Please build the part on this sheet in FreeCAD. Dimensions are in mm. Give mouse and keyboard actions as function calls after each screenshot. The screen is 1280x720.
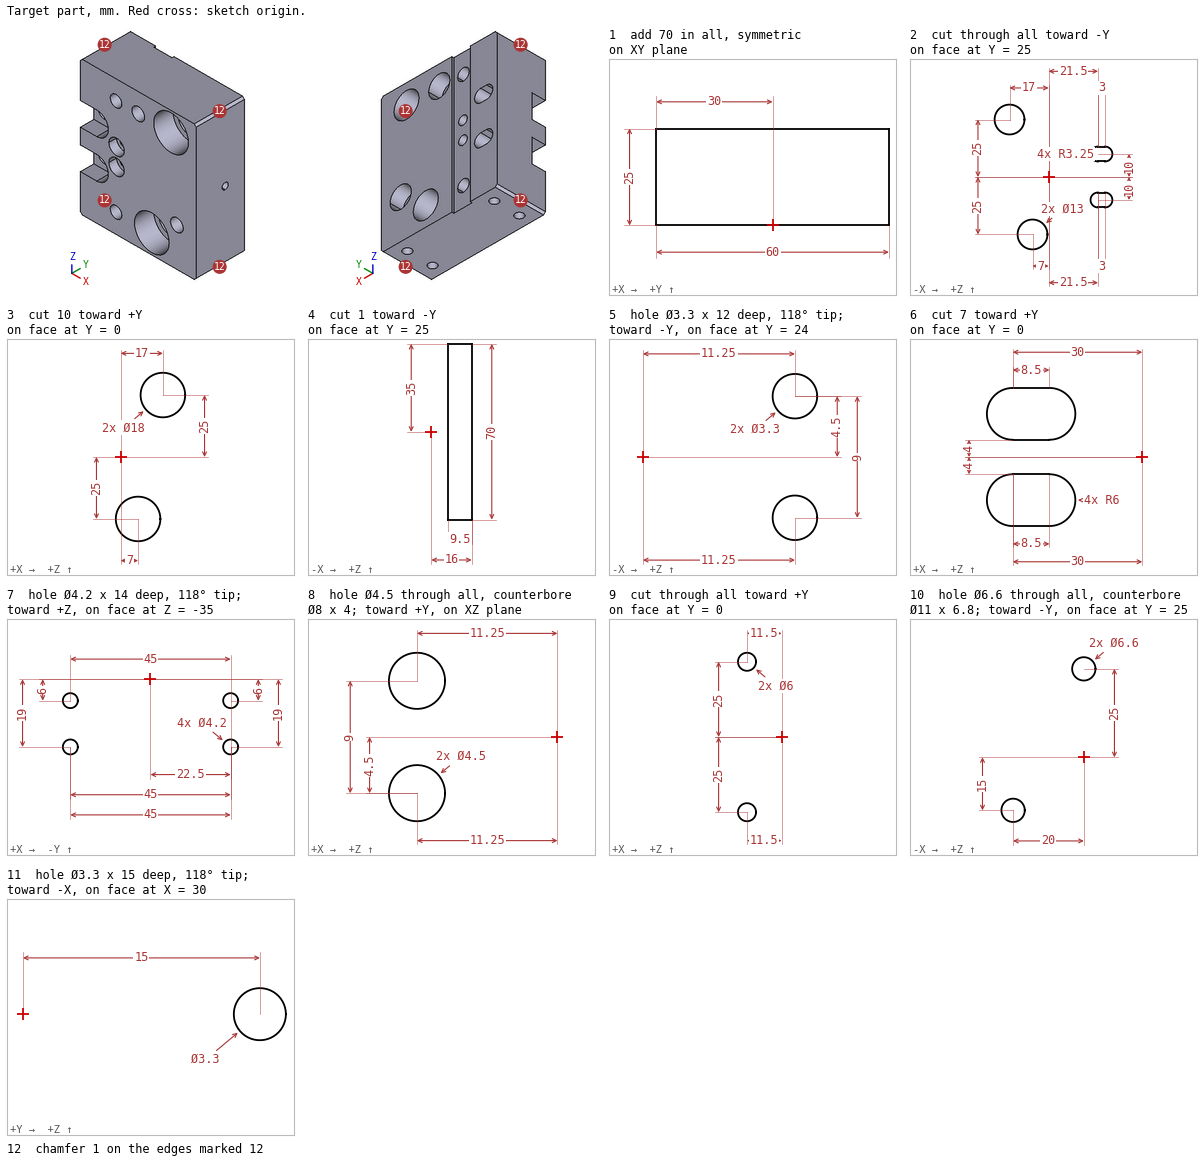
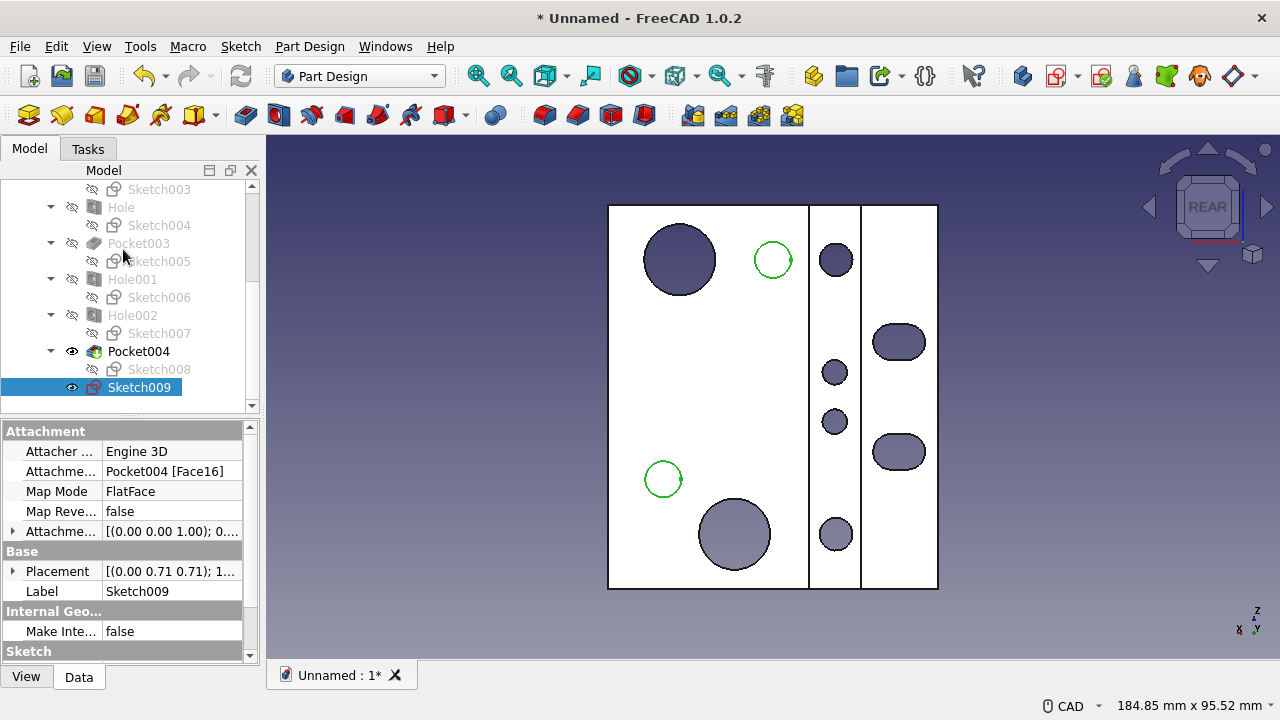
click(279, 116)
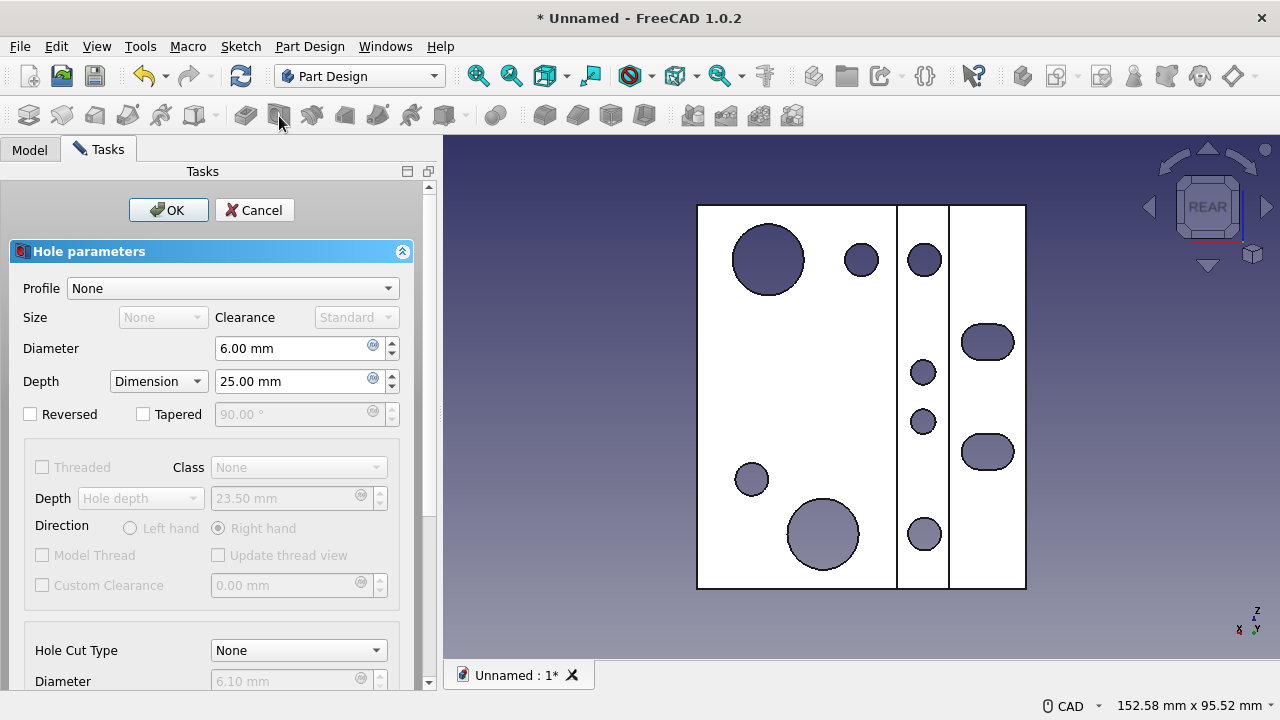
triple_click(300, 348)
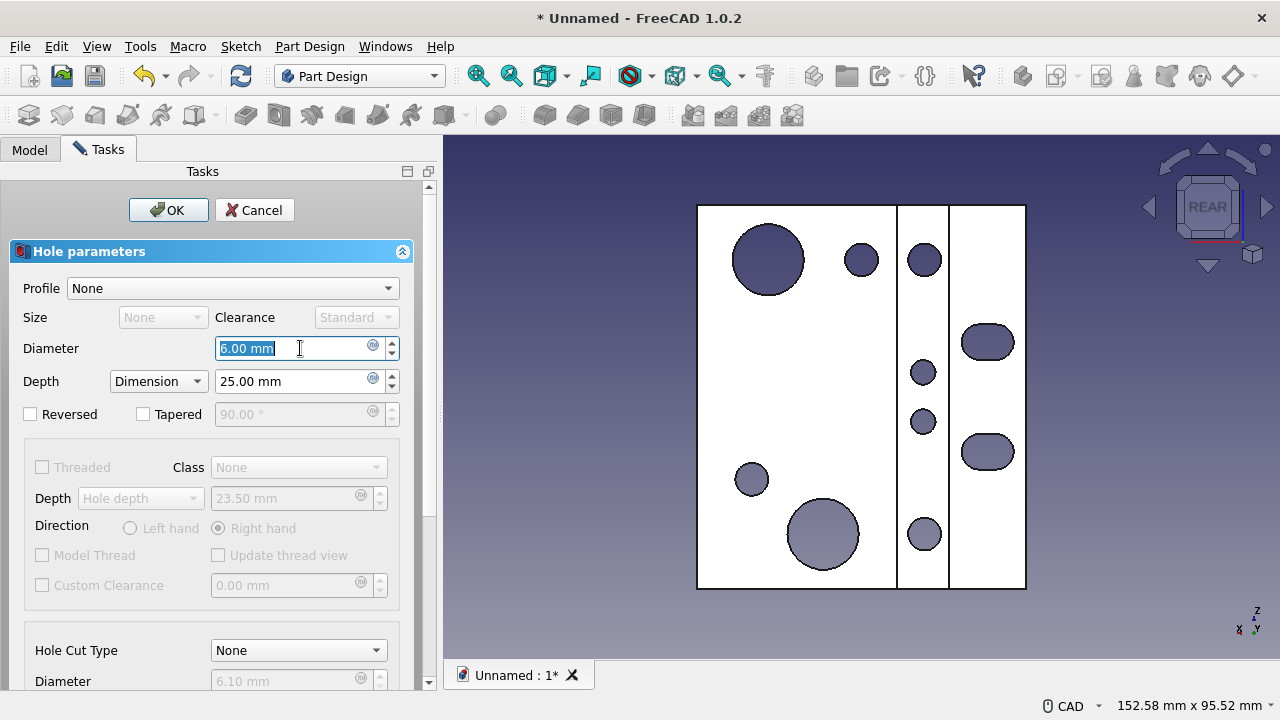
text(6.6)
key(Tab)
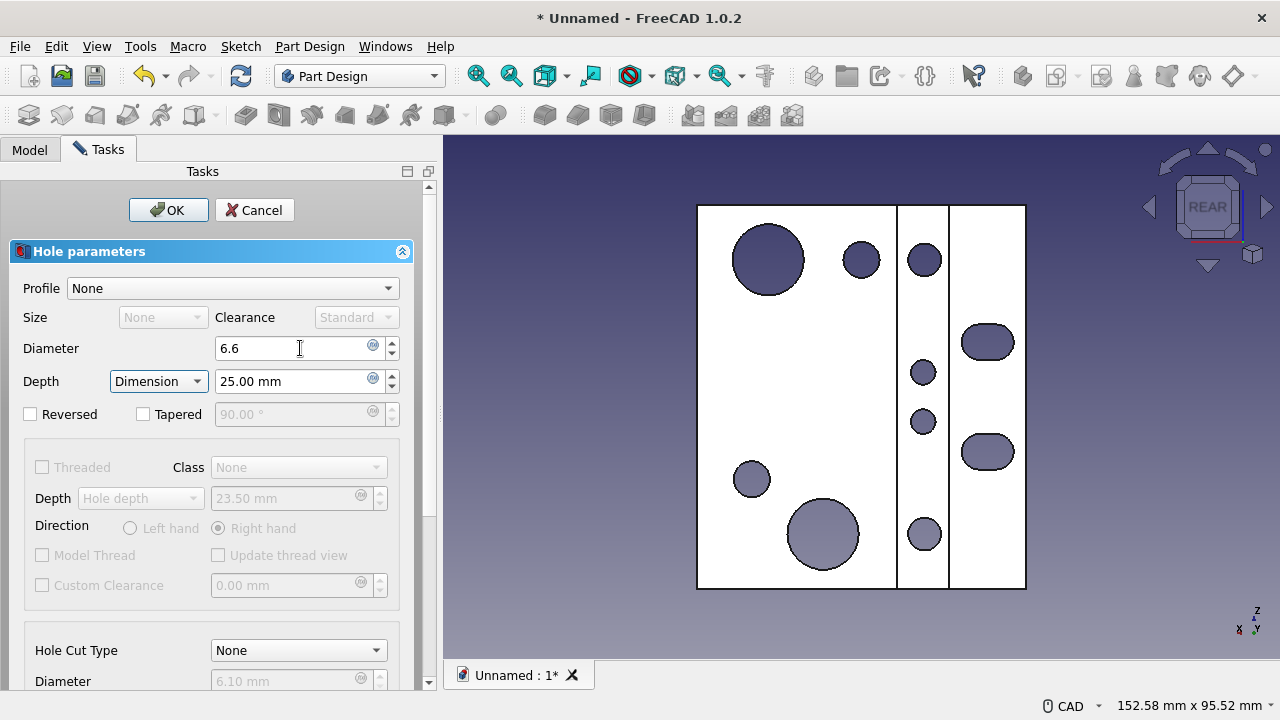
click(160, 382)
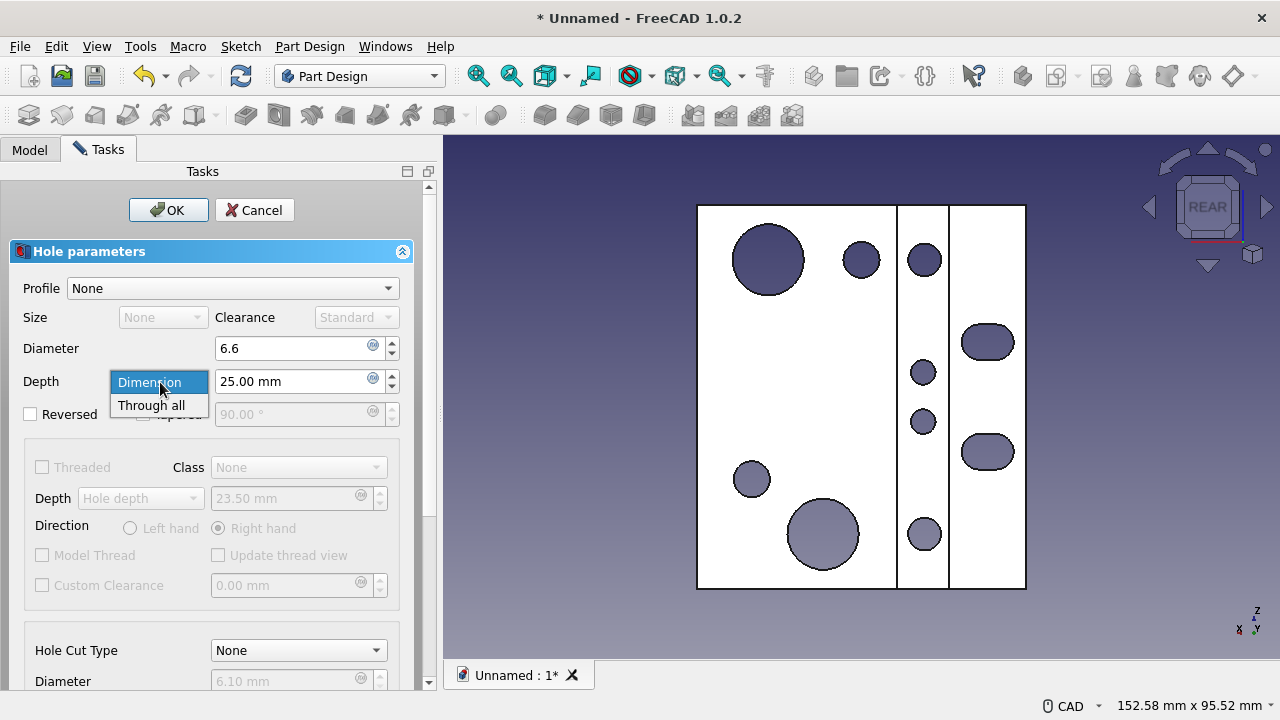
click(158, 406)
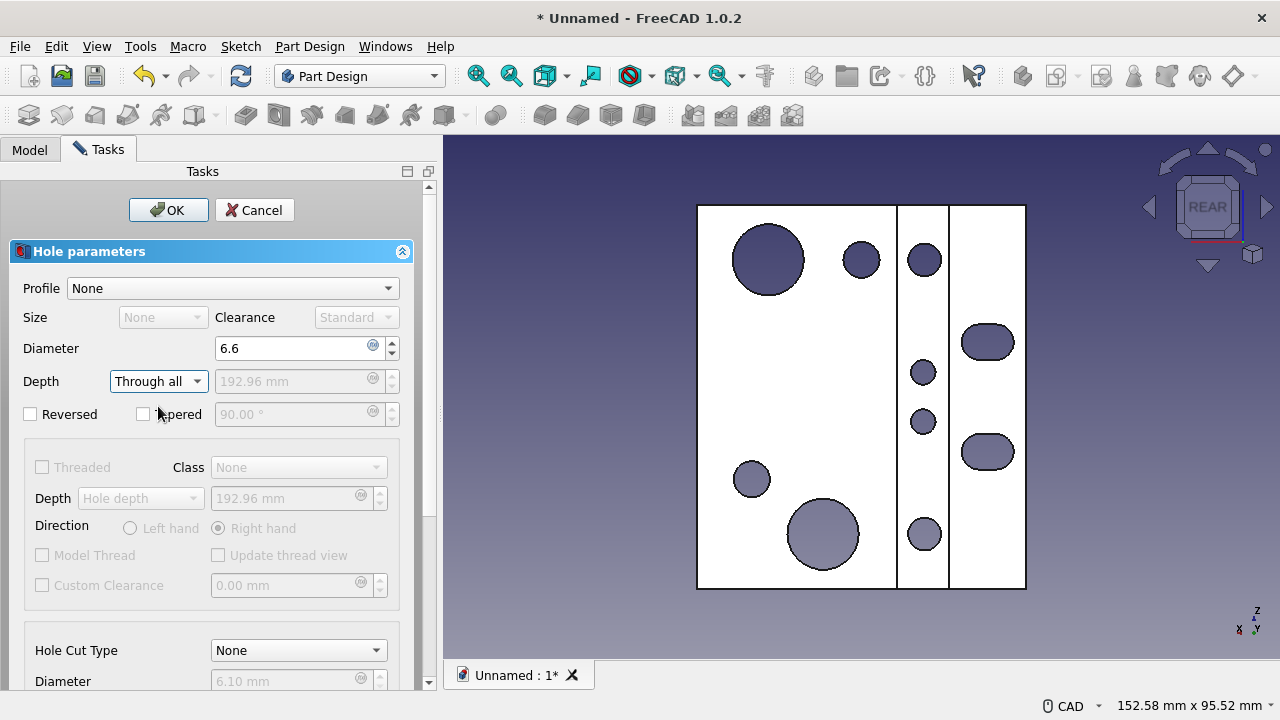
click(300, 650)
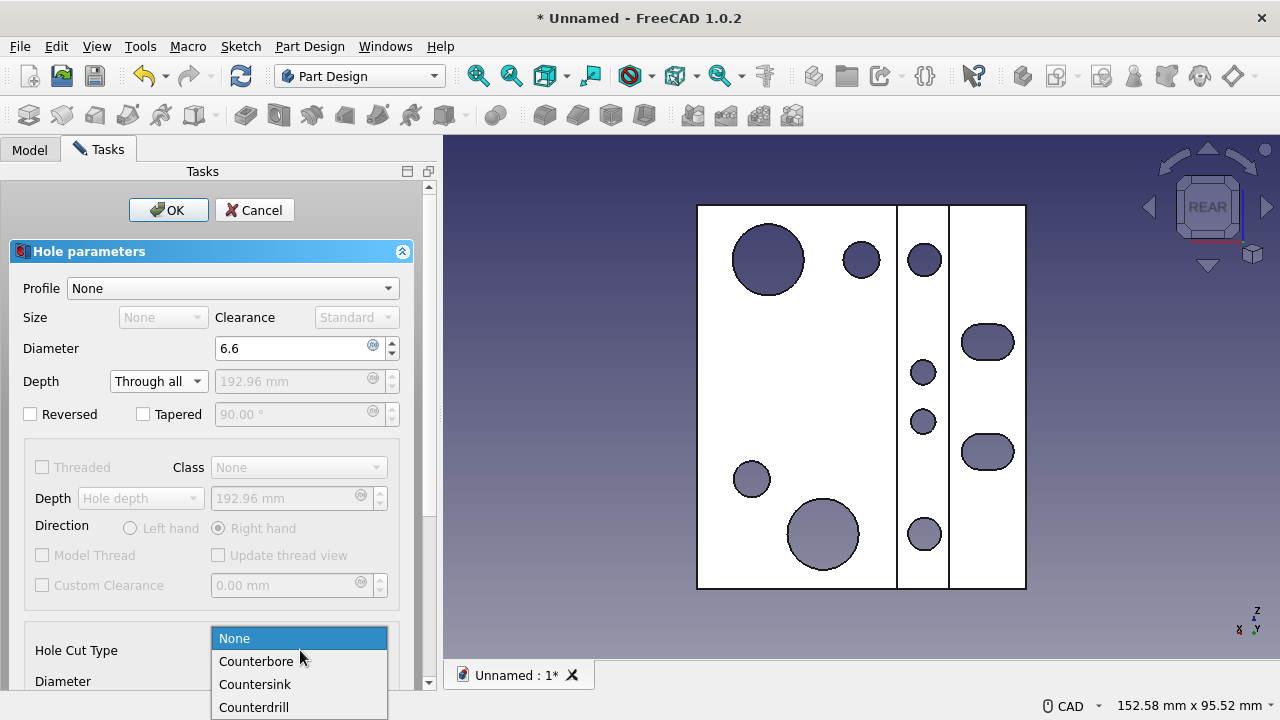
click(298, 662)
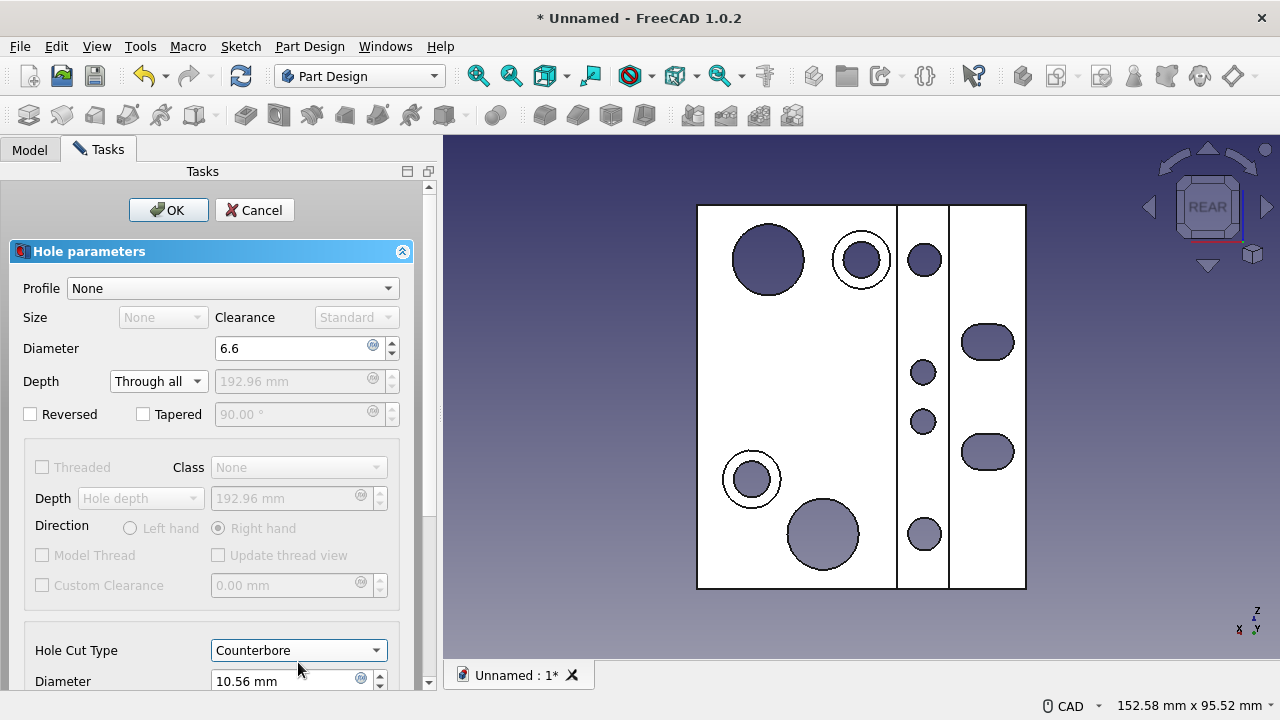
scroll(429, 436, down, 2)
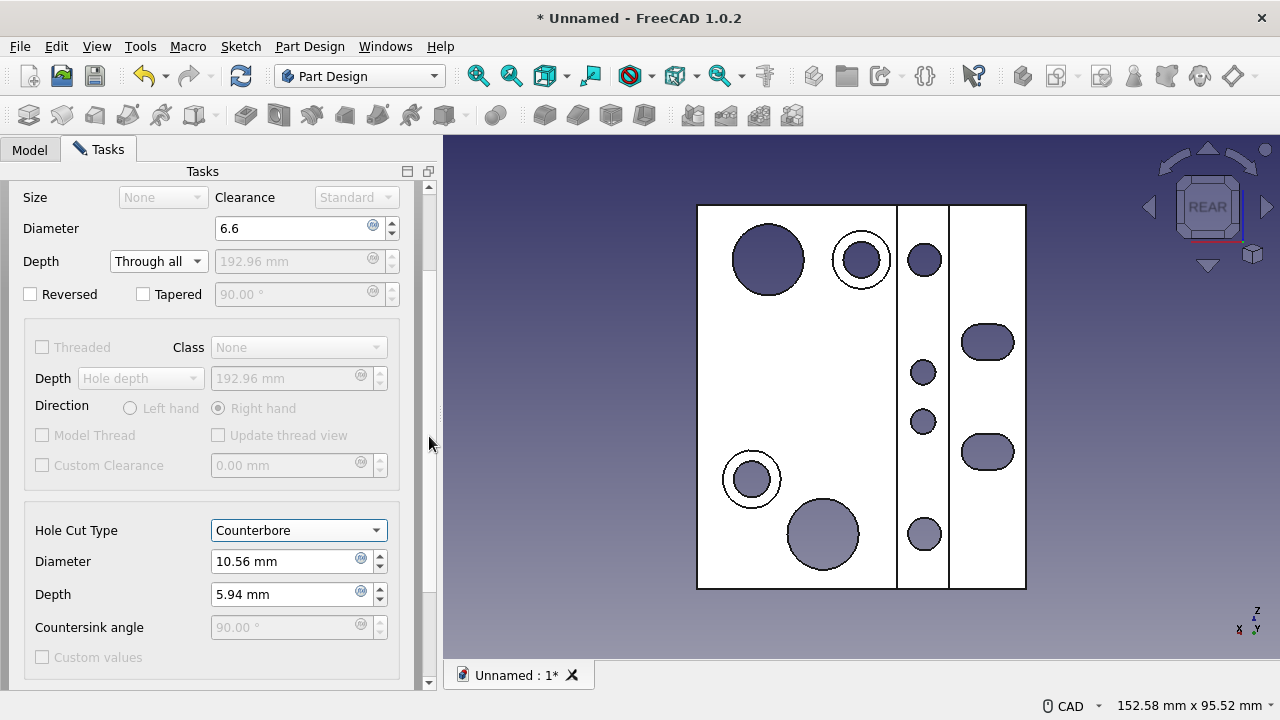
triple_click(292, 562)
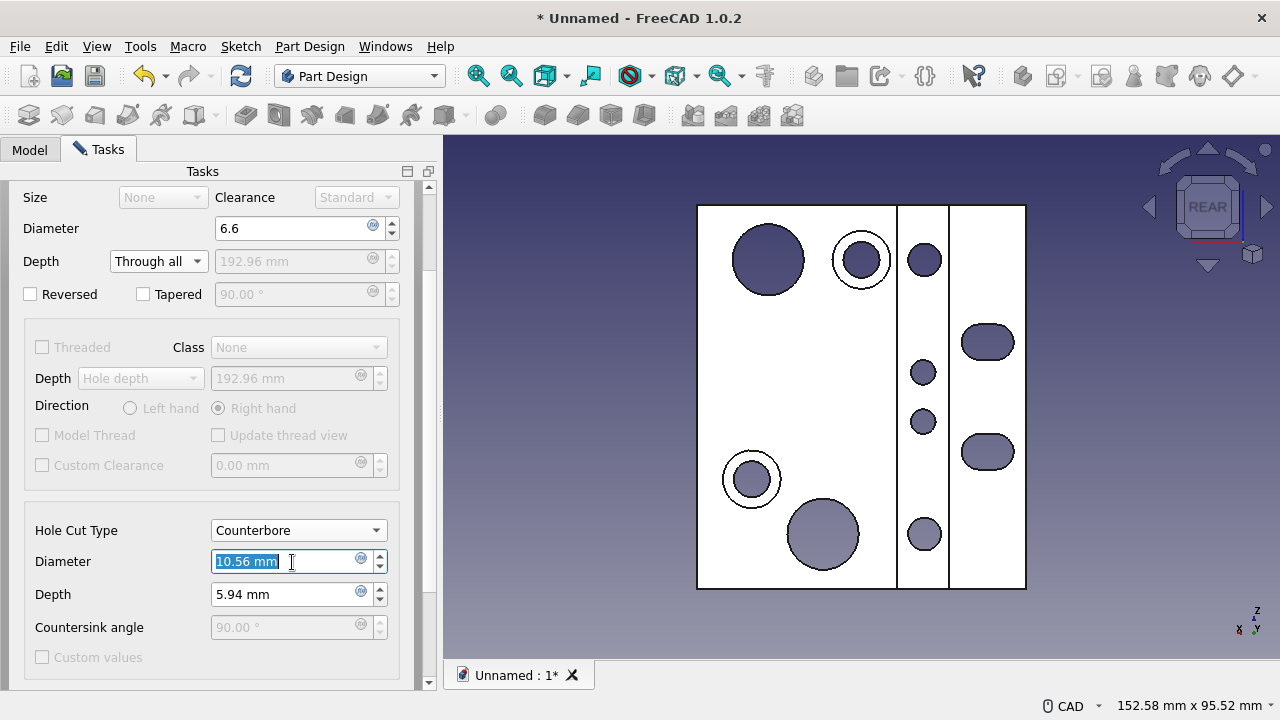
text(11)
key(Tab)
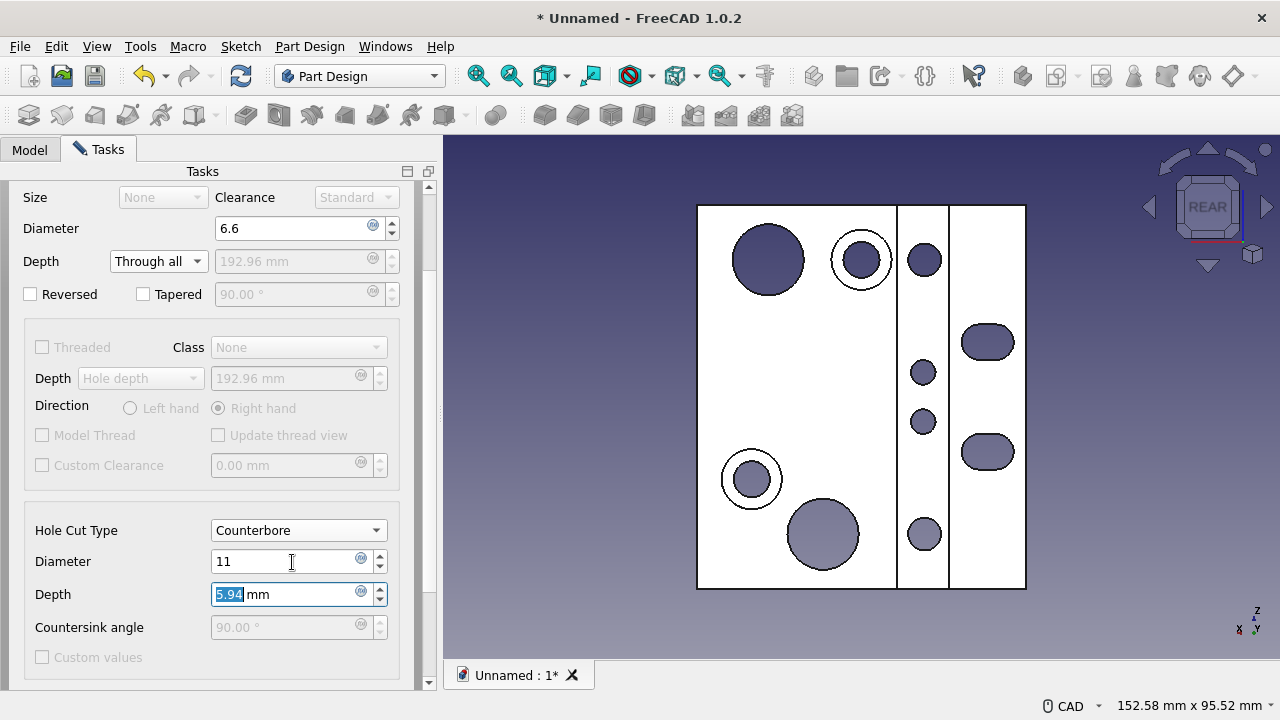
text(6.8)
key(Tab)